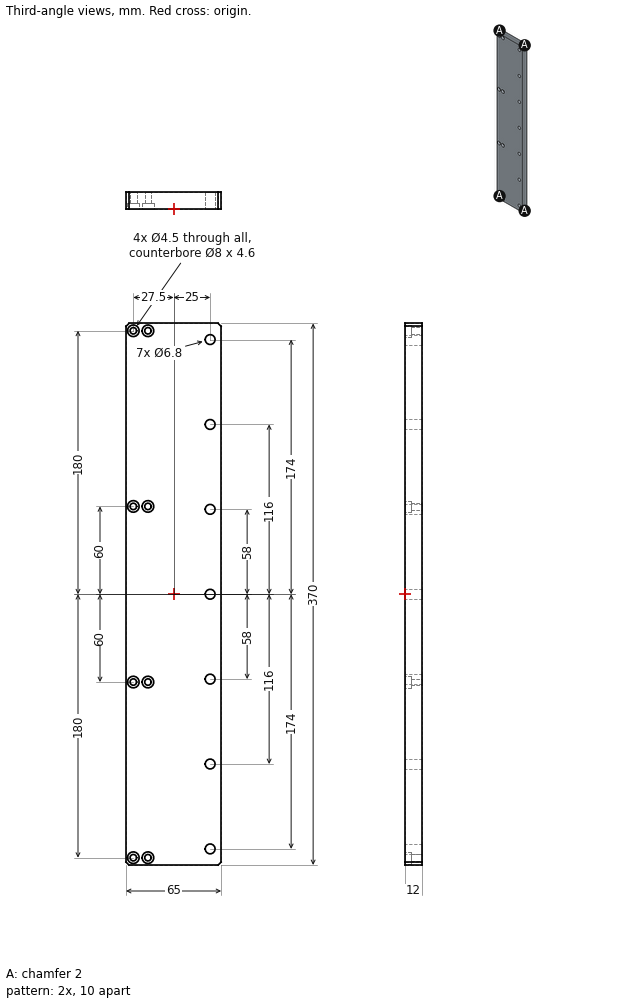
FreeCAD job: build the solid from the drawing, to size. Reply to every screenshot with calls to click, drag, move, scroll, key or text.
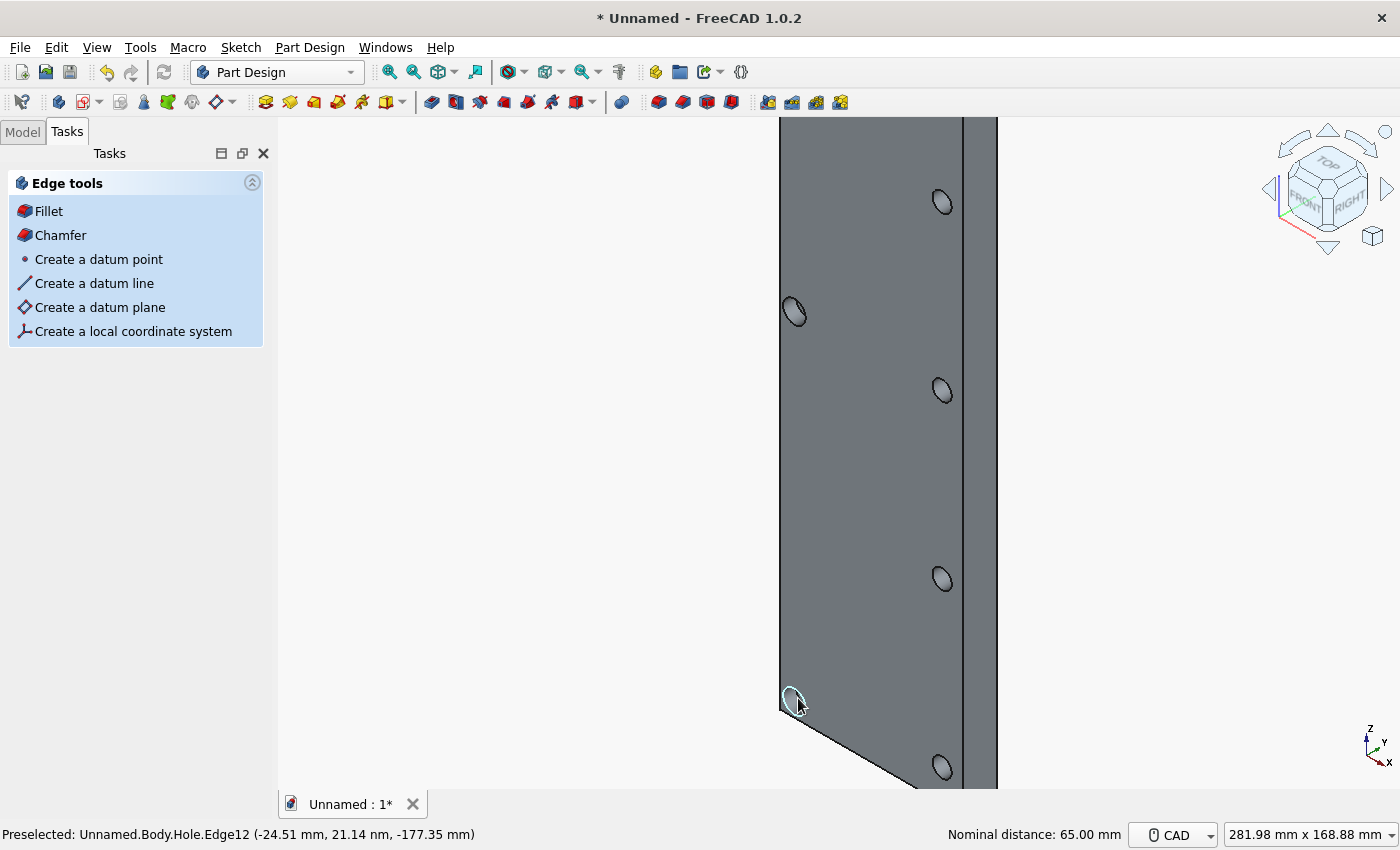
key(v)
key(f)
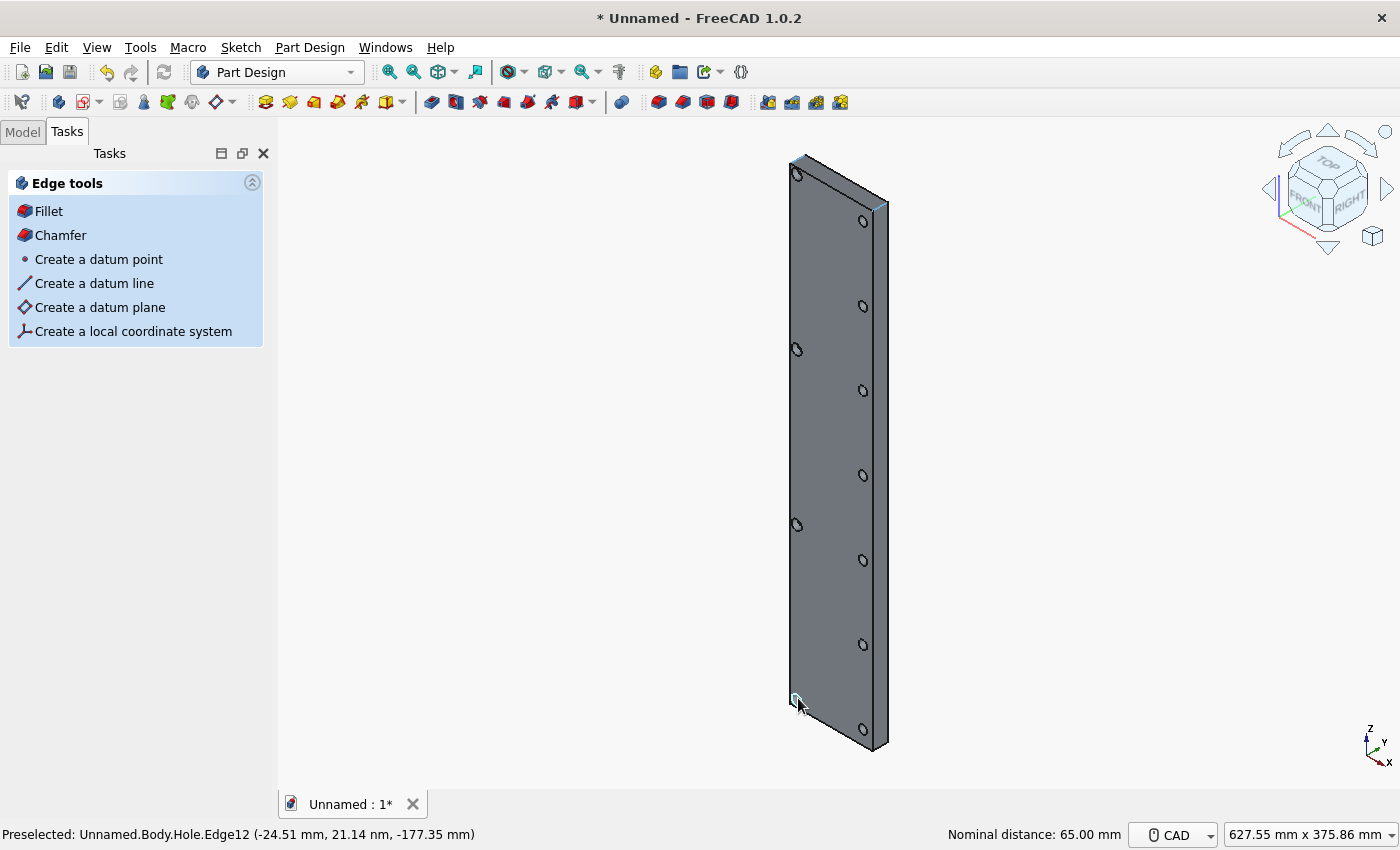
key(1)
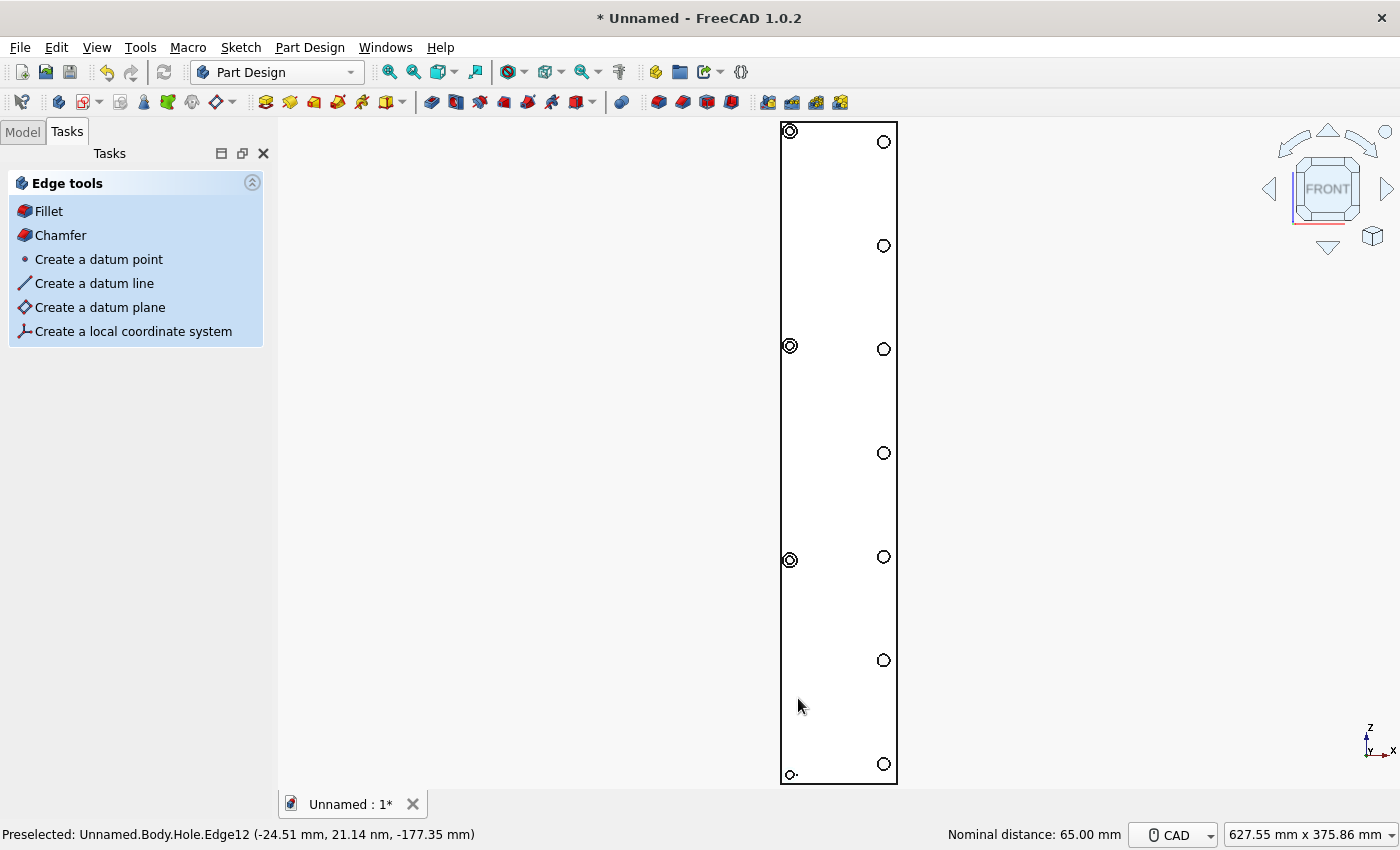
key(3)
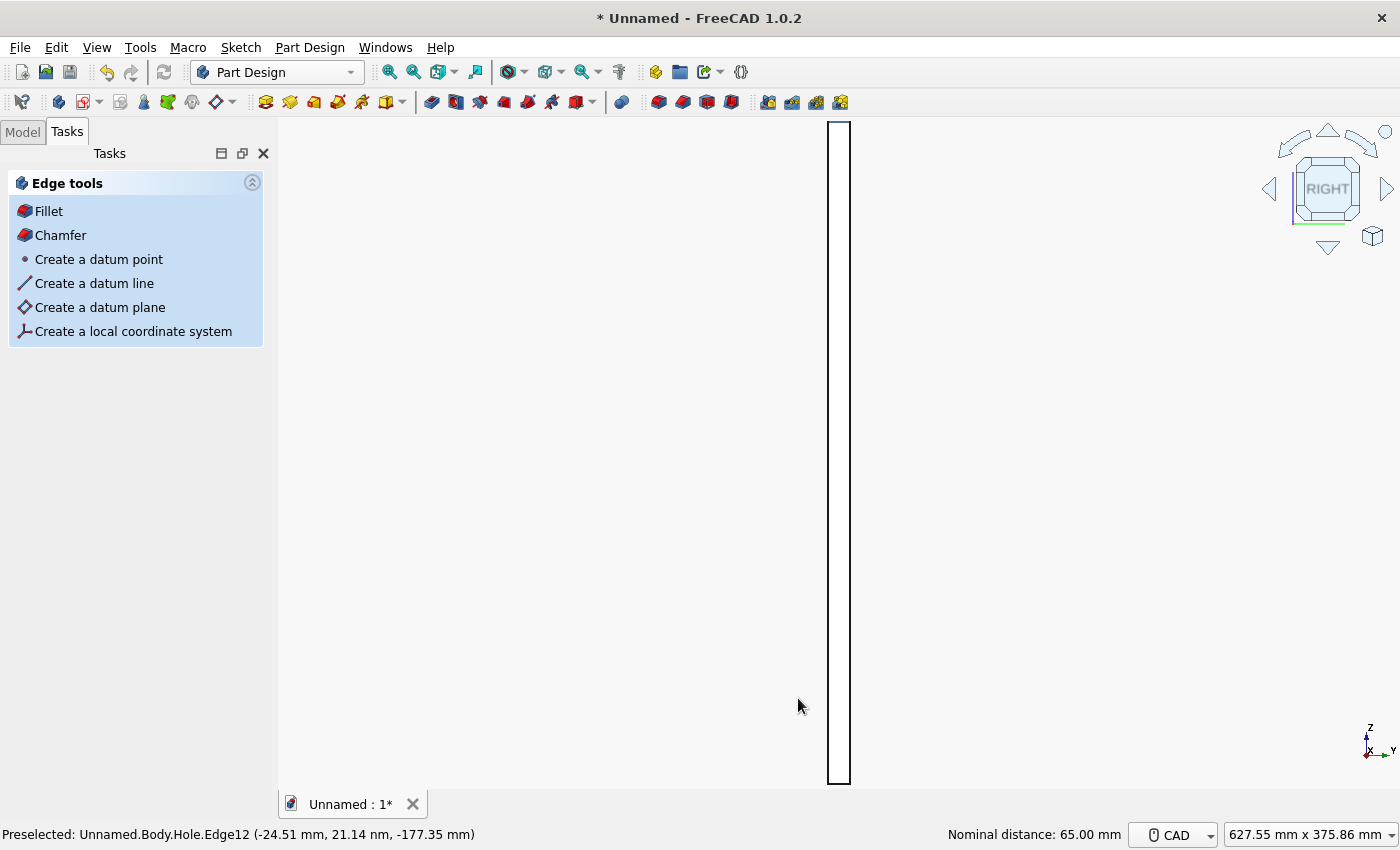
key(5)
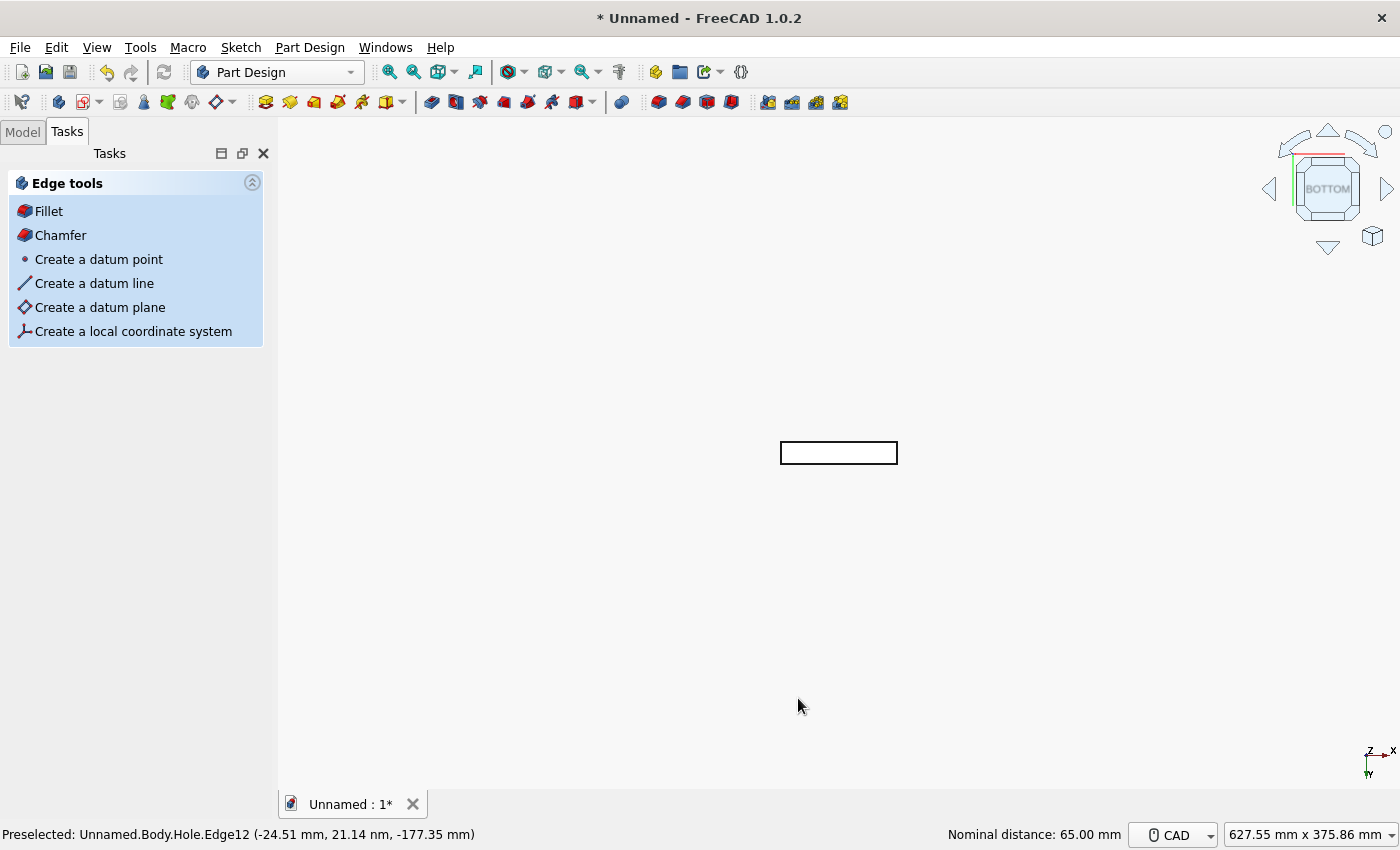
click(390, 72)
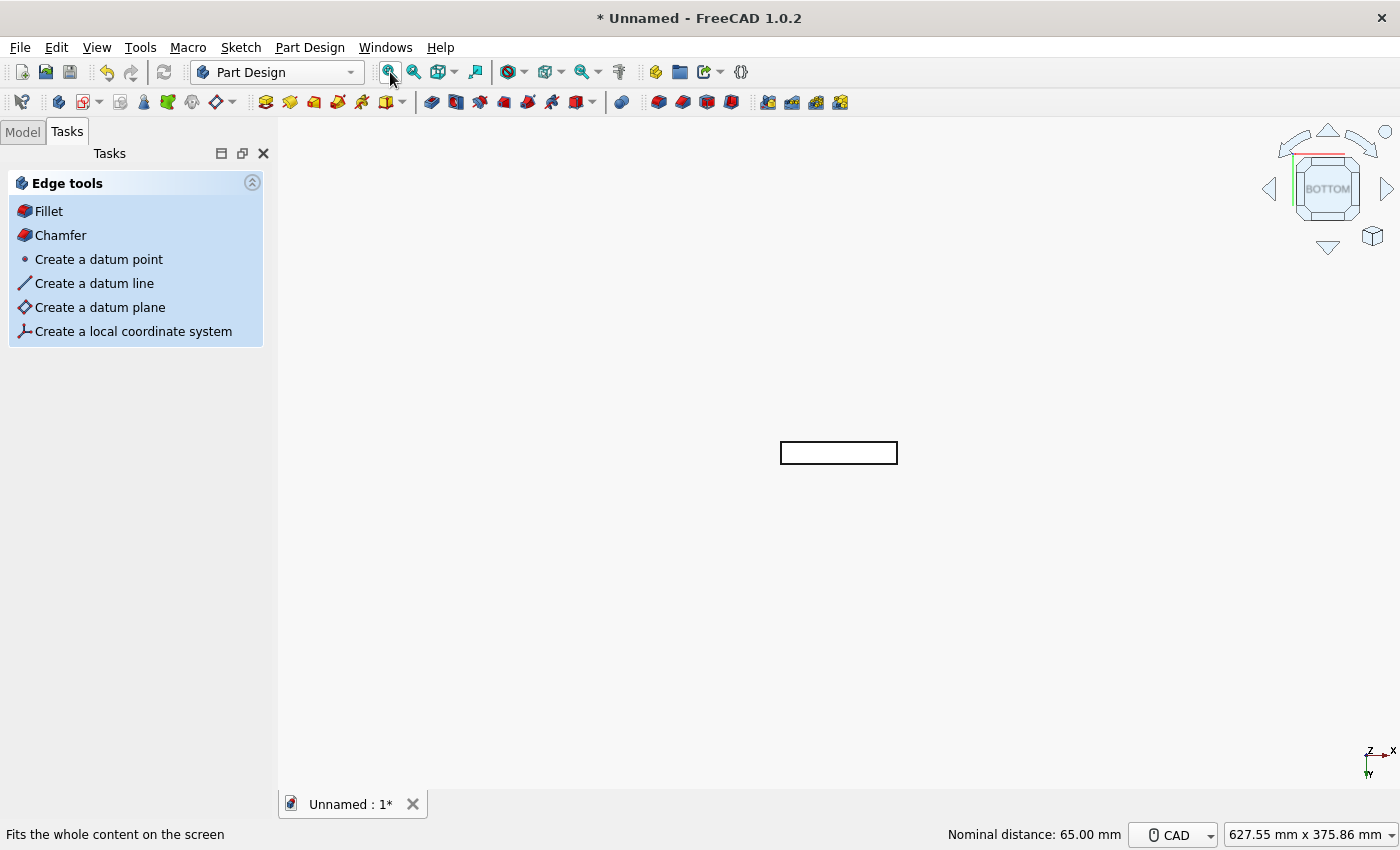
click(781, 452, ctrl)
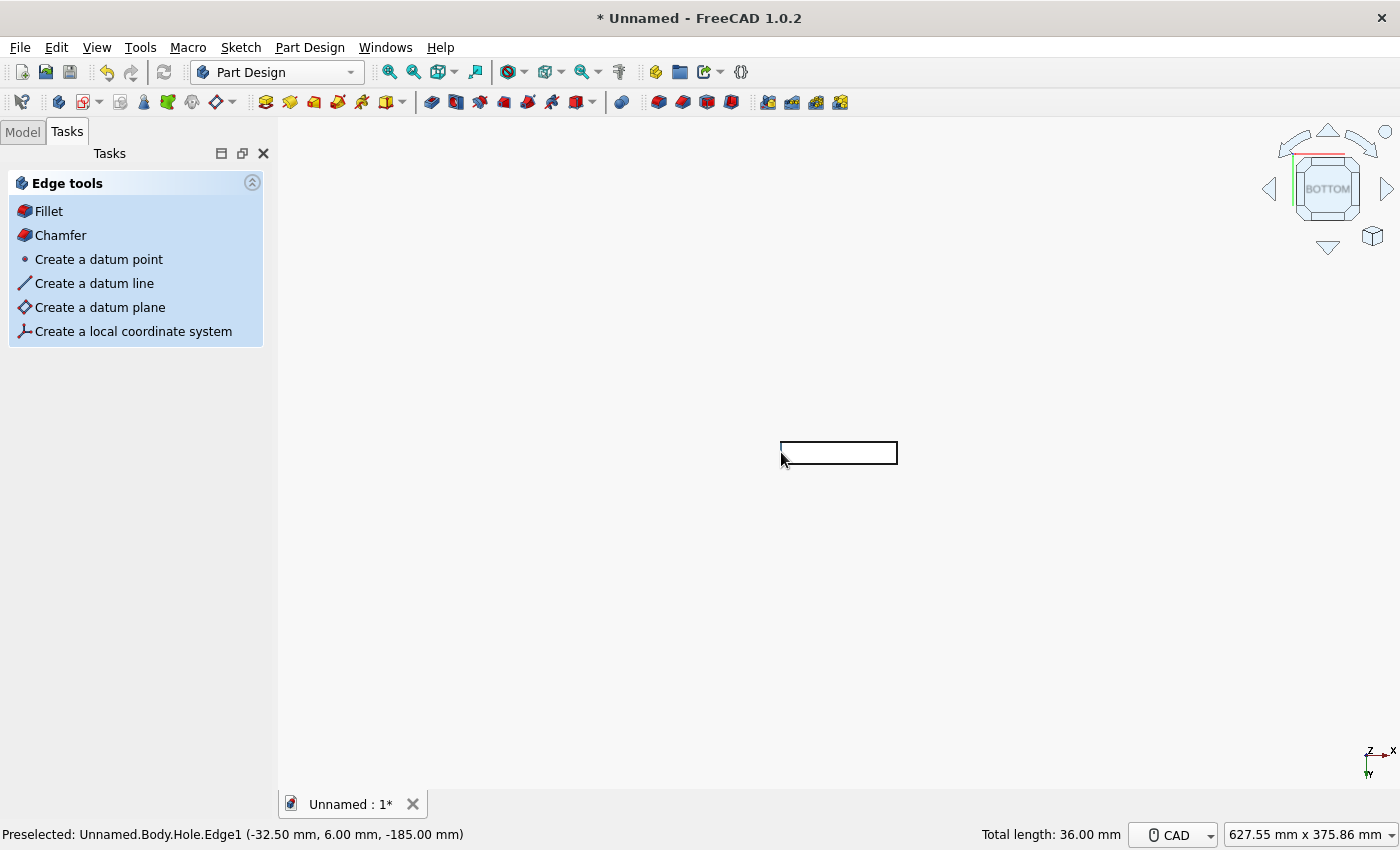
click(897, 452, ctrl)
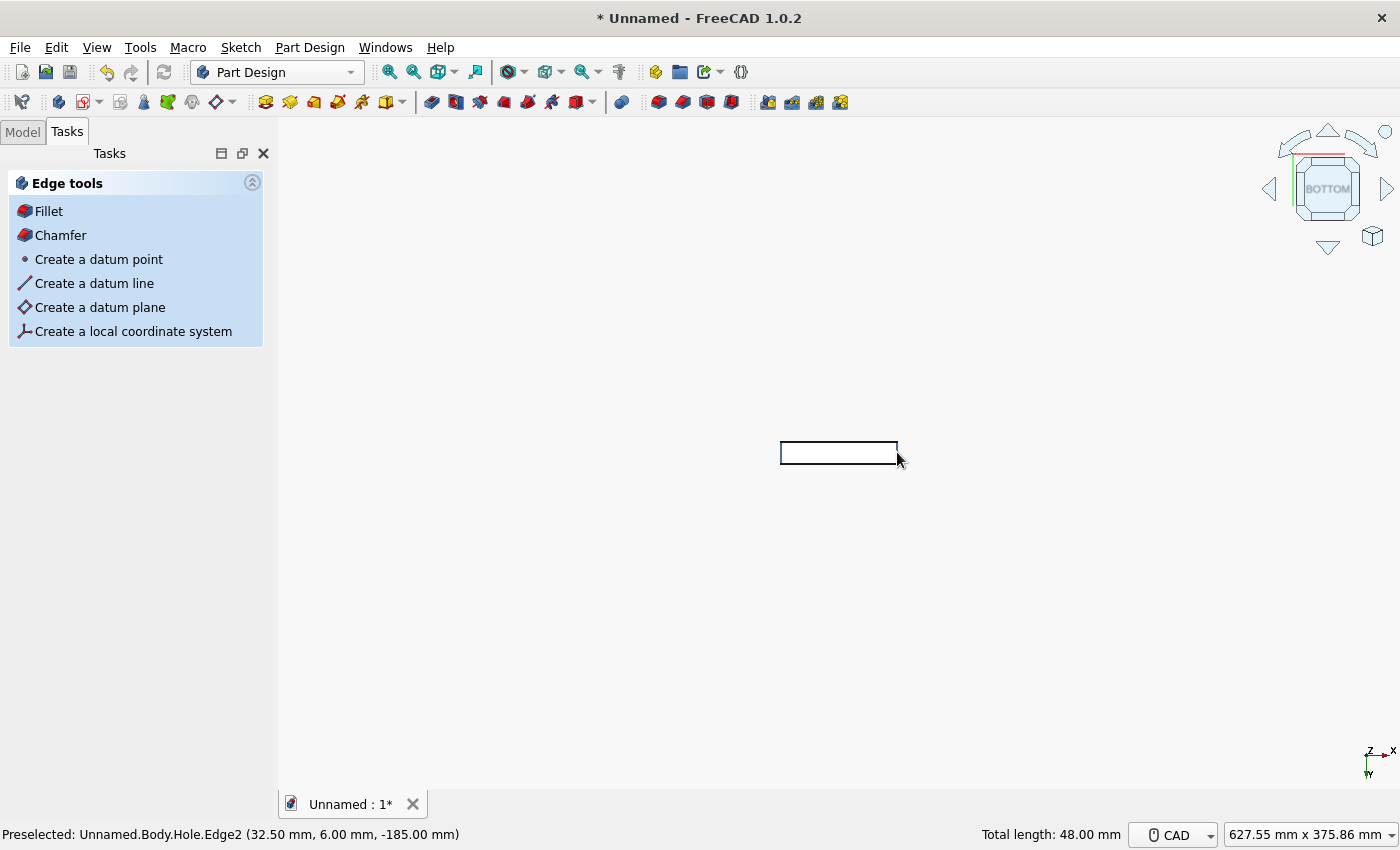
click(684, 102)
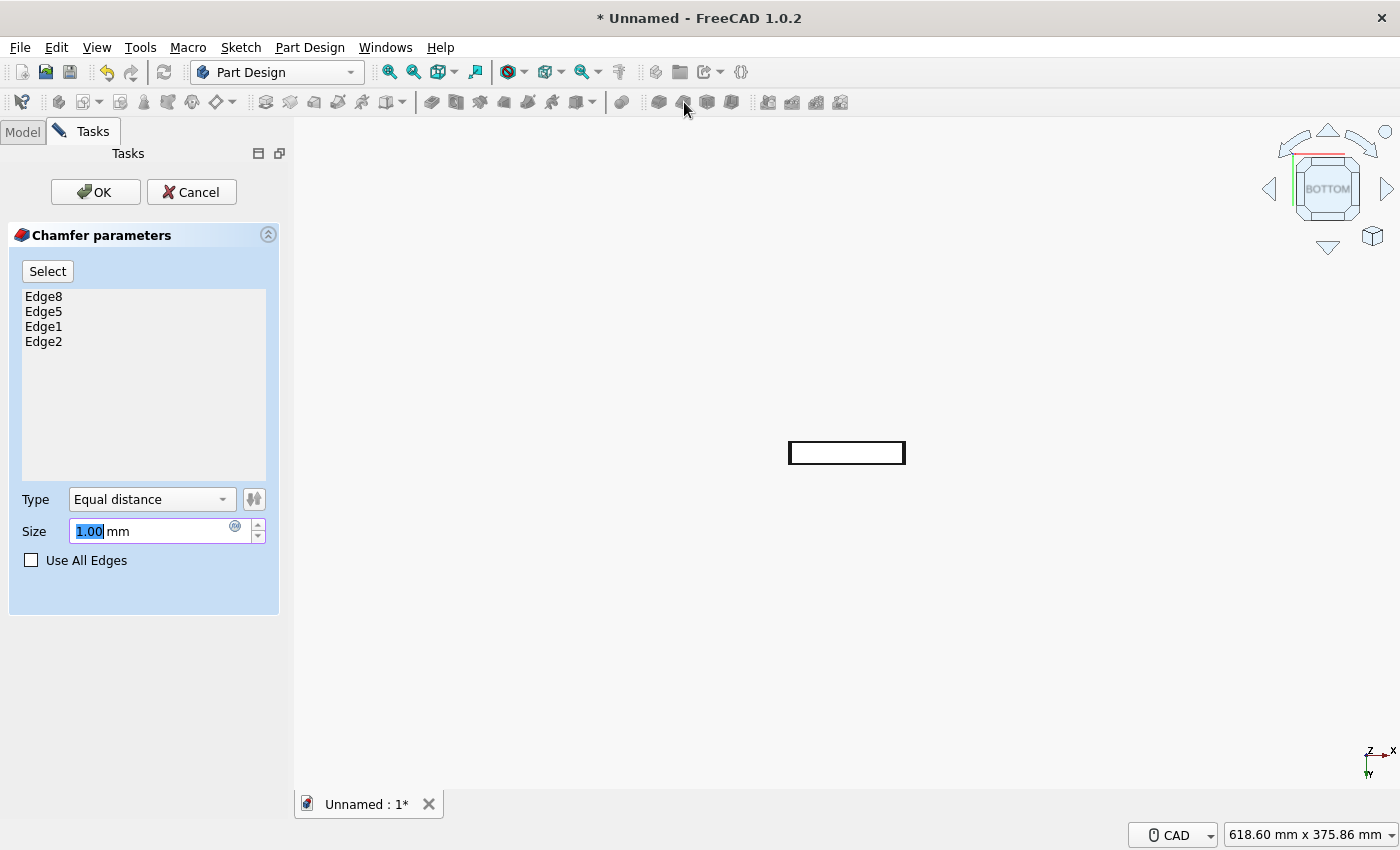
text(2)
key(Tab)